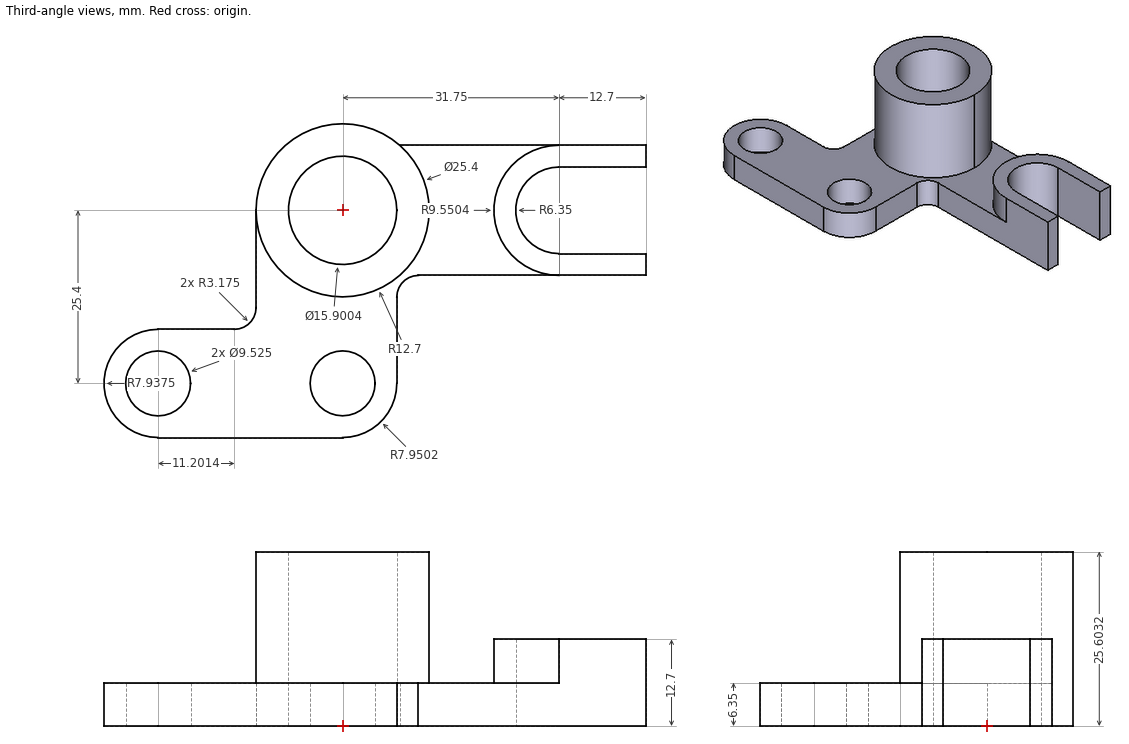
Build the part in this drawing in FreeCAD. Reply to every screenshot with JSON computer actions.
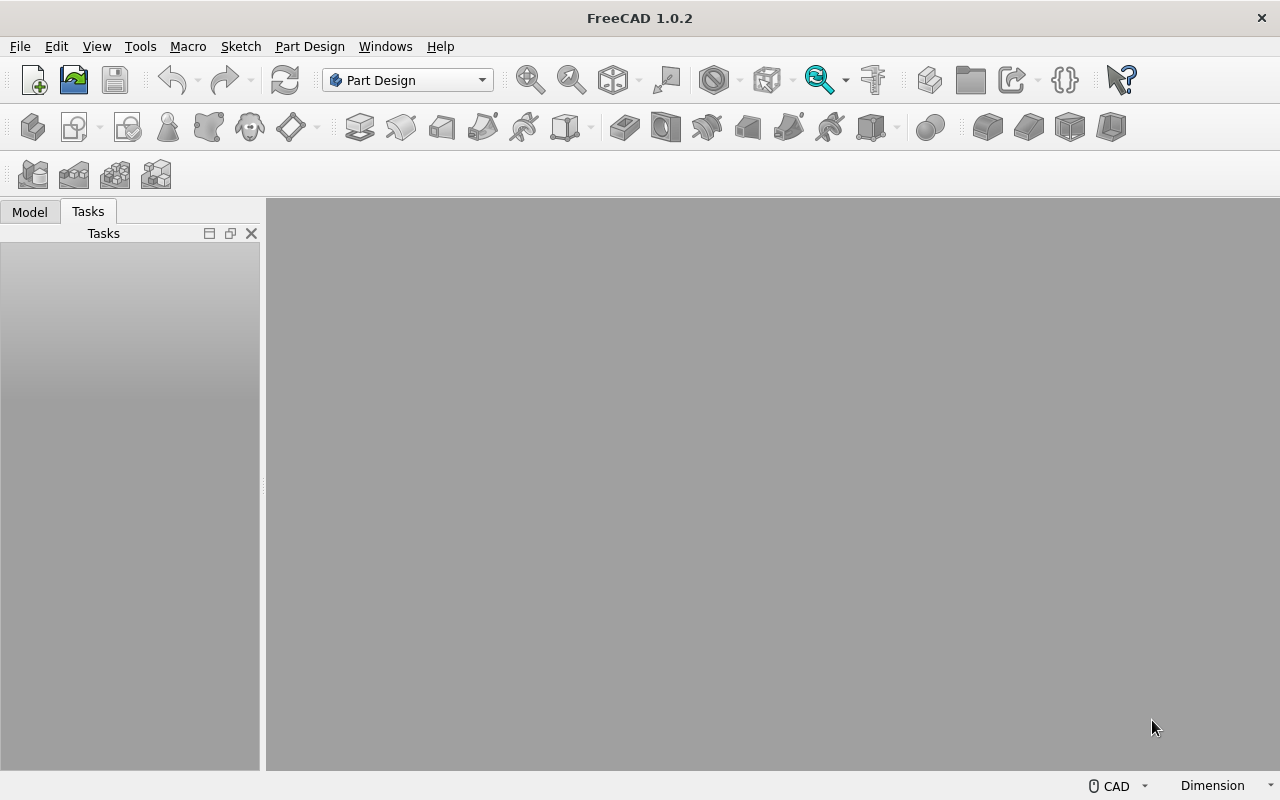
{"action": "left_click", "coordinate": [33, 80]}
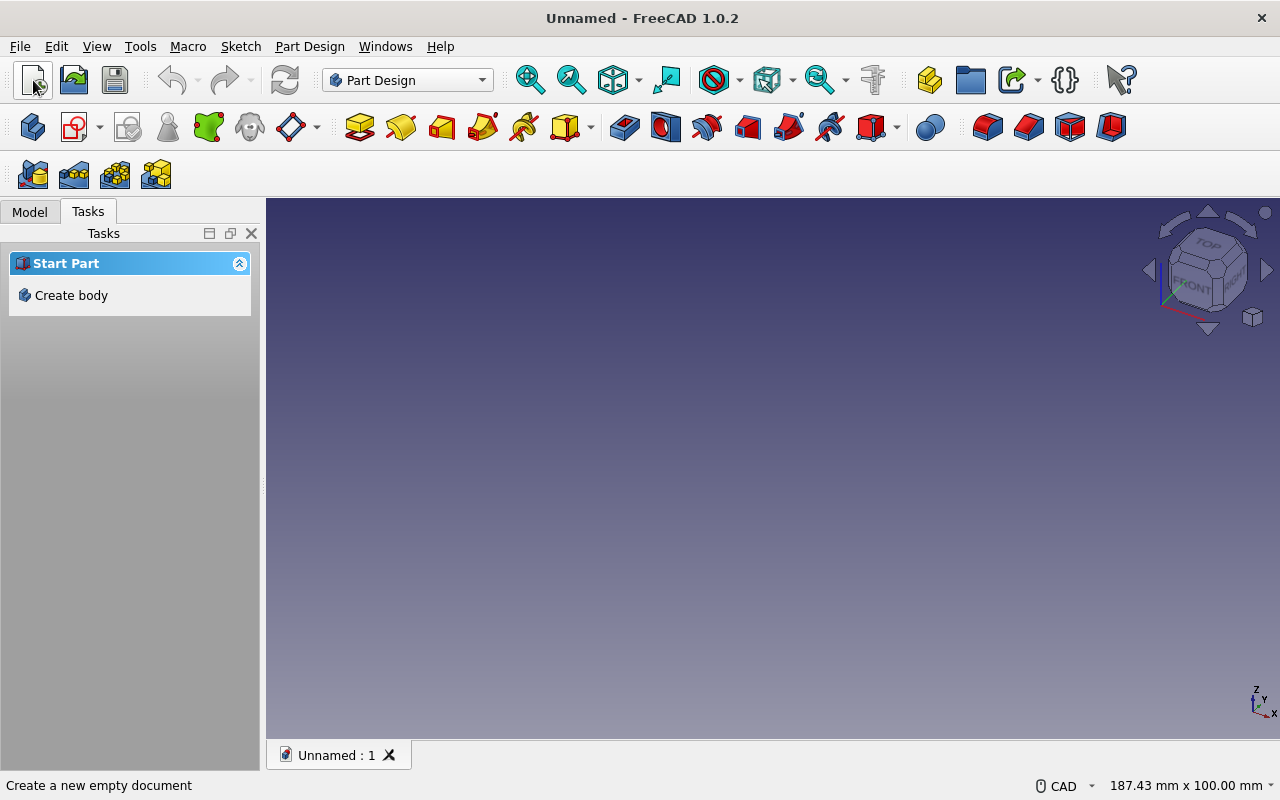
{"action": "left_click", "coordinate": [74, 128]}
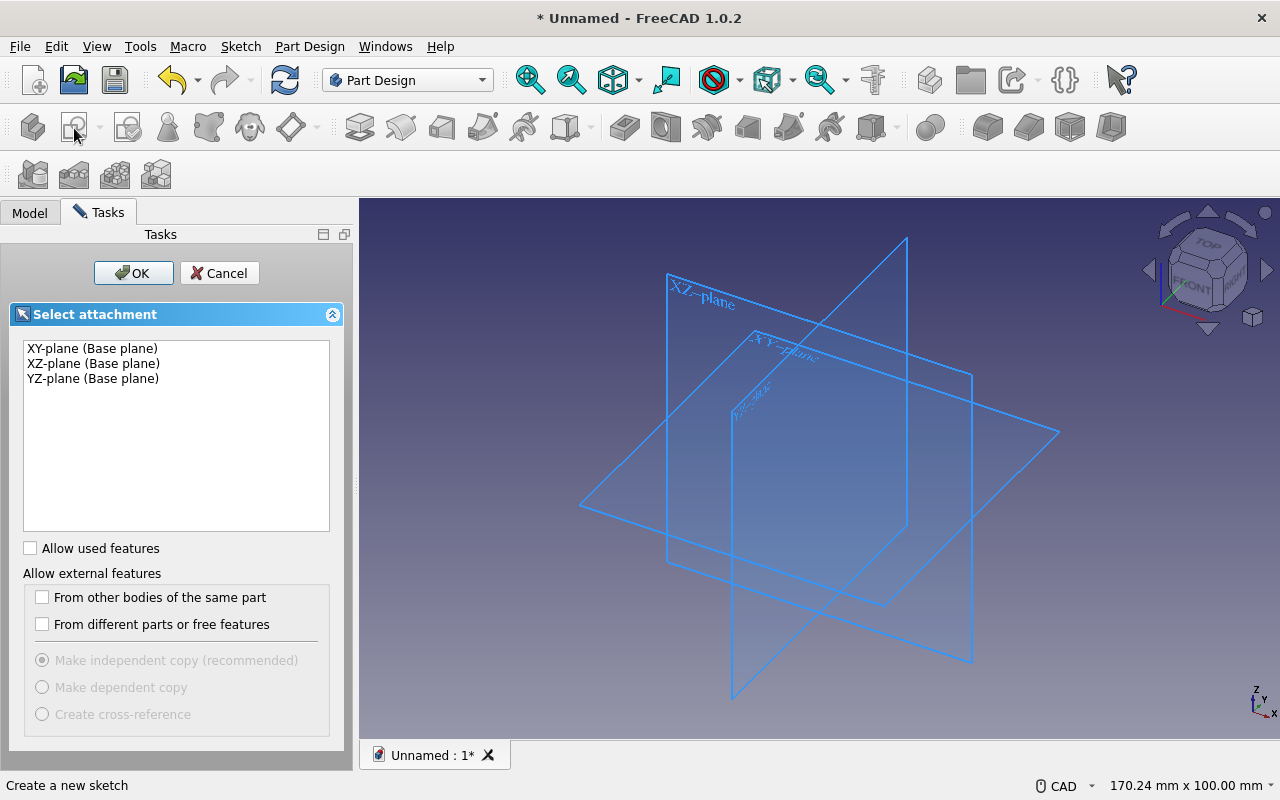
{"action": "left_click", "coordinate": [84, 348]}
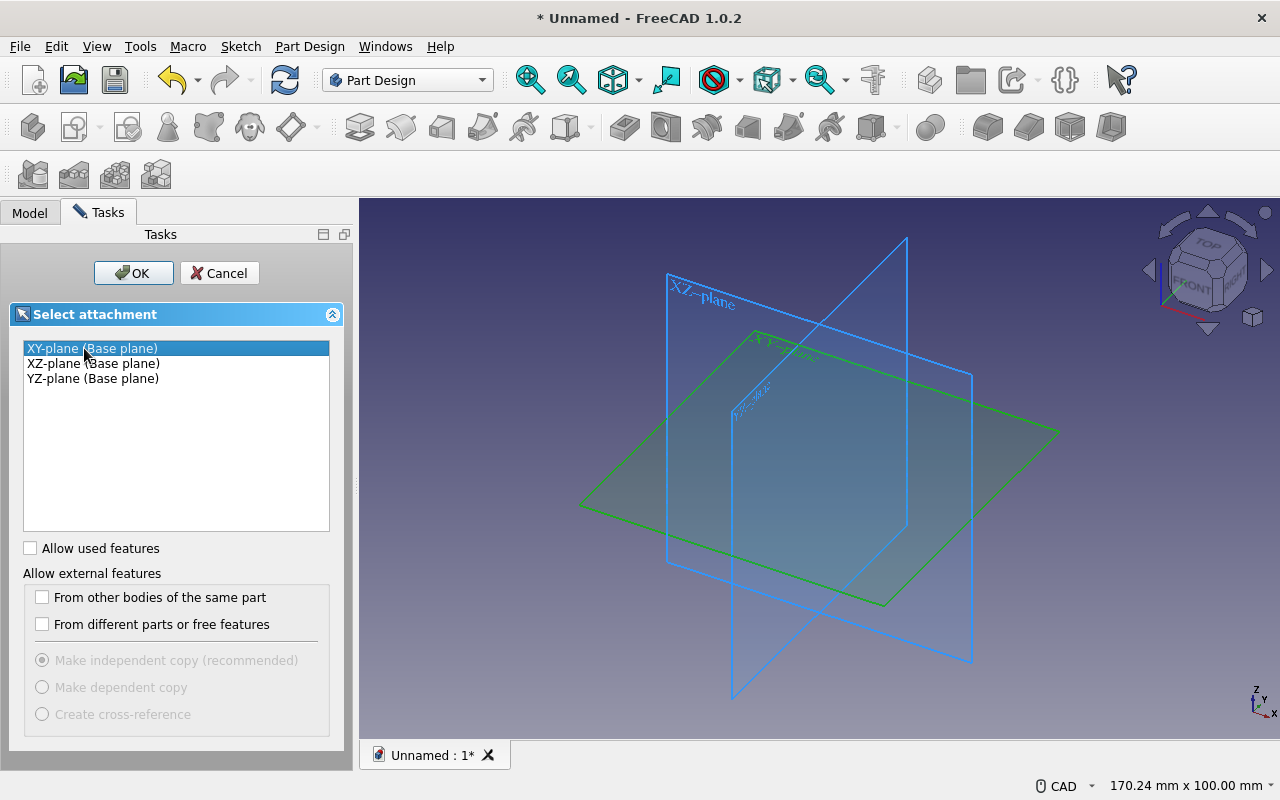
{"action": "left_click", "coordinate": [134, 273]}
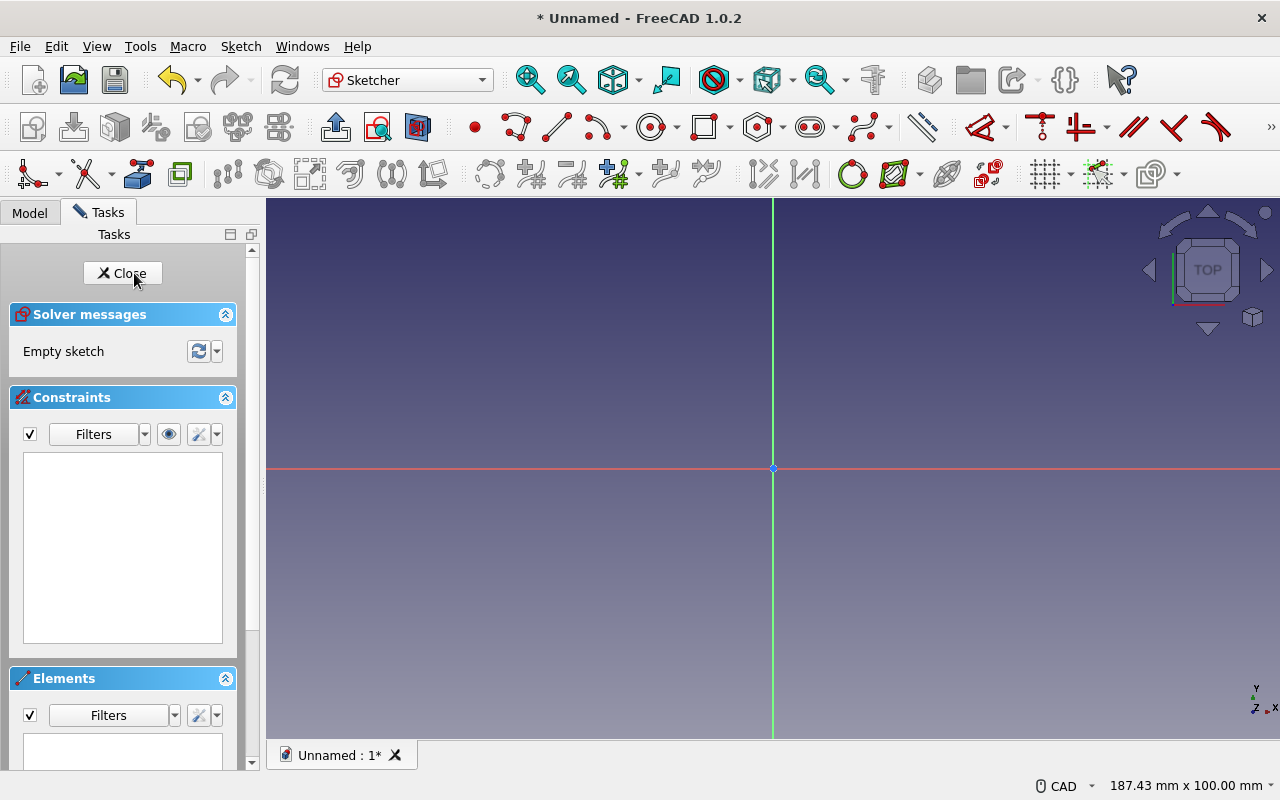
{"action": "scroll", "coordinate": [813, 468], "scroll_direction": "up", "scroll_amount": 5}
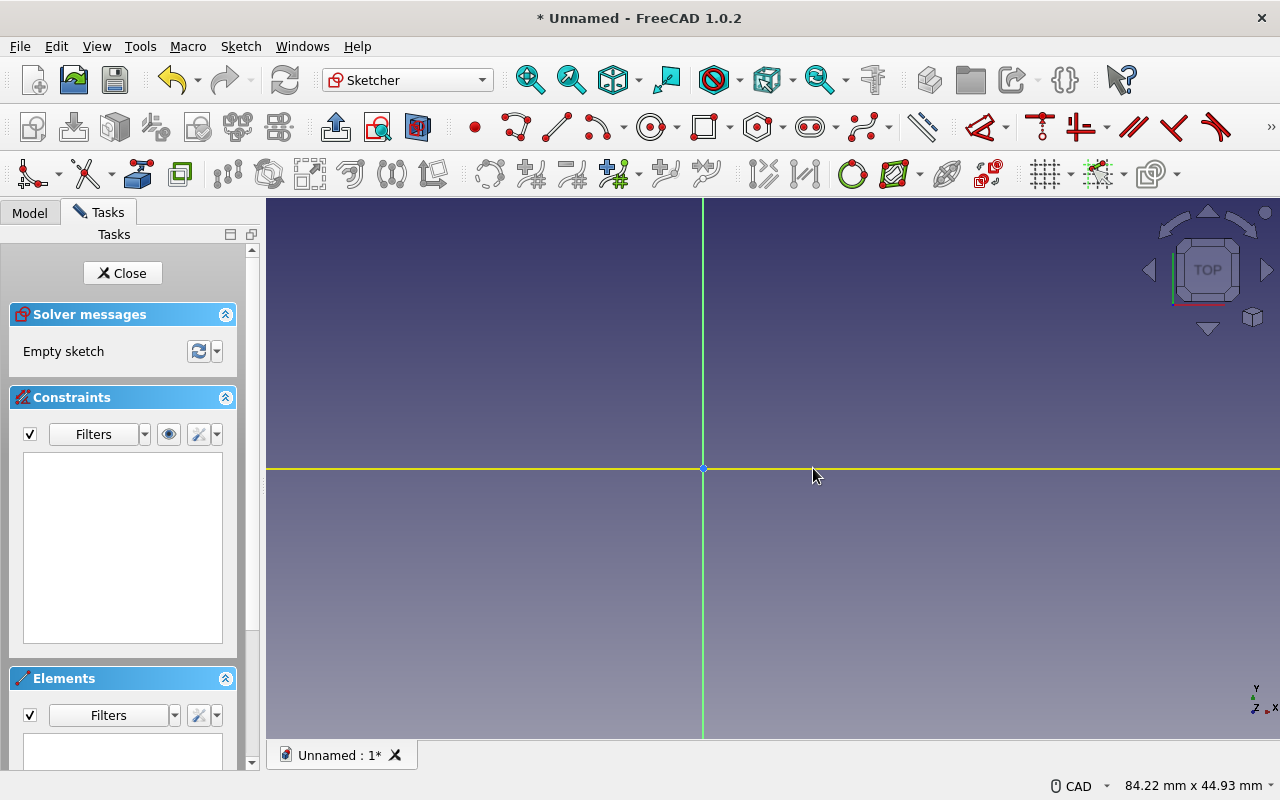
{"action": "left_click", "coordinate": [650, 128]}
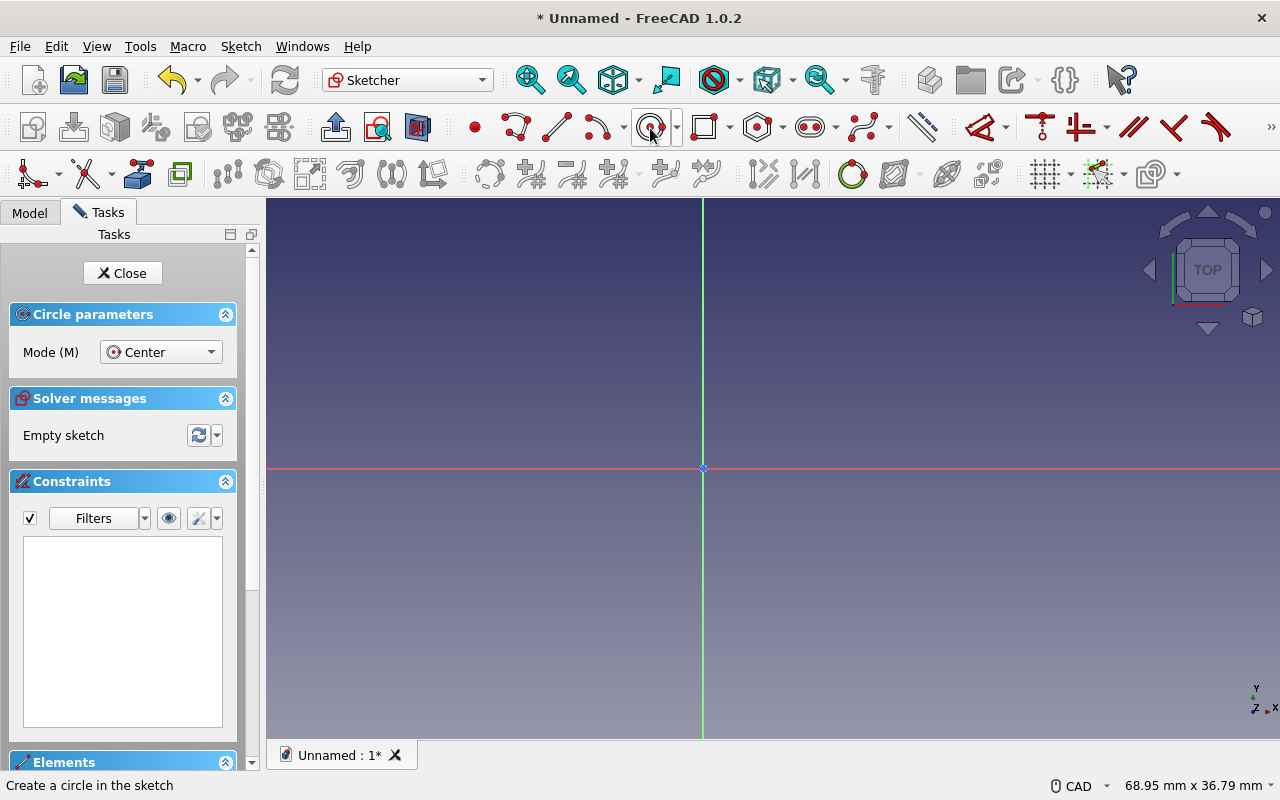
{"action": "left_click", "coordinate": [703, 468]}
{"action": "left_click", "coordinate": [835, 336]}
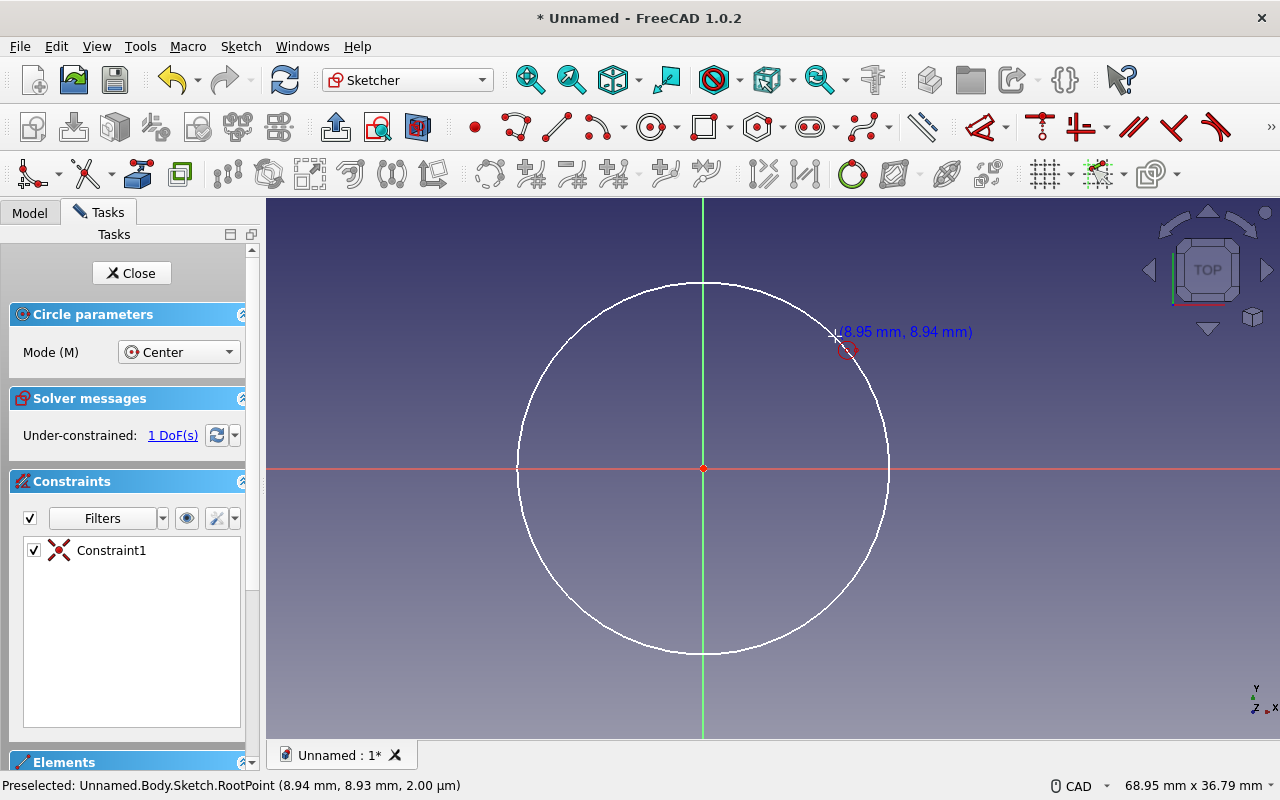
{"action": "left_click", "coordinate": [703, 468]}
{"action": "left_click", "coordinate": [786, 386]}
{"action": "key", "text": "Escape"}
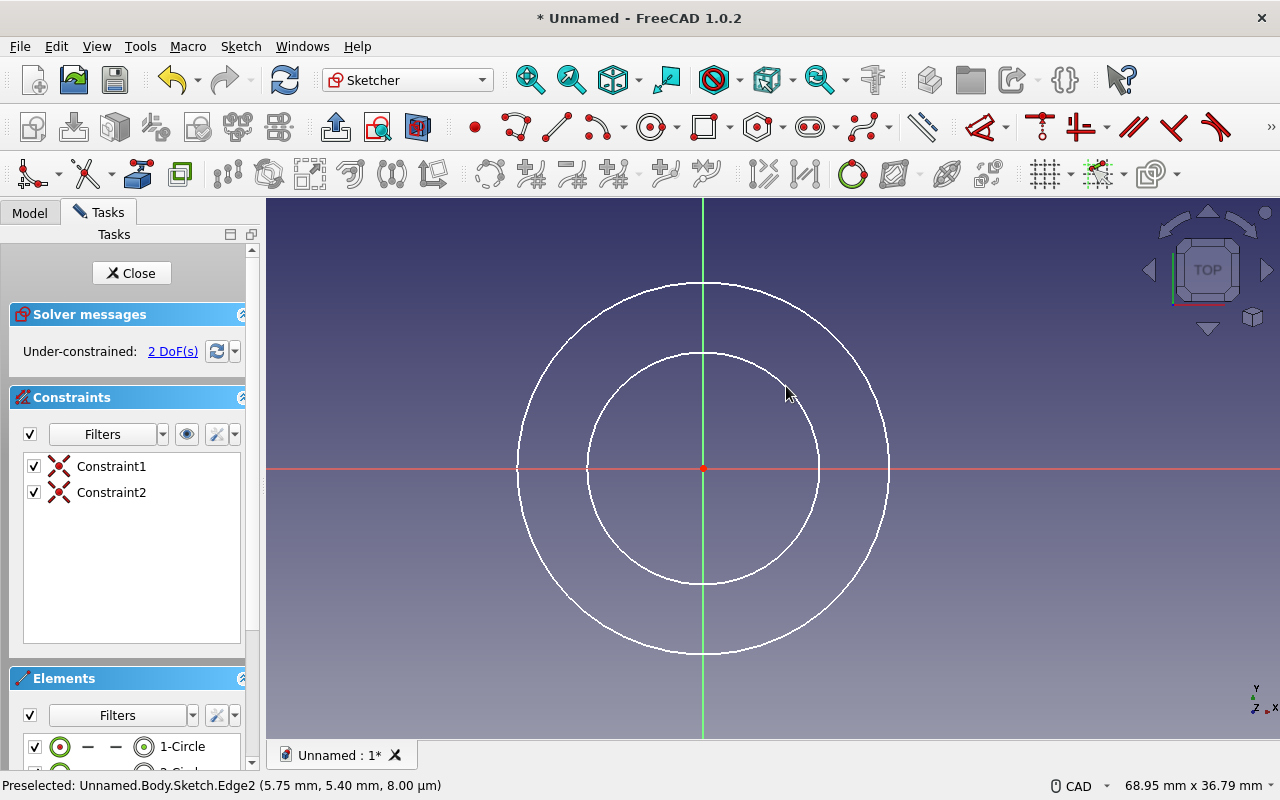
{"action": "left_click", "coordinate": [980, 128]}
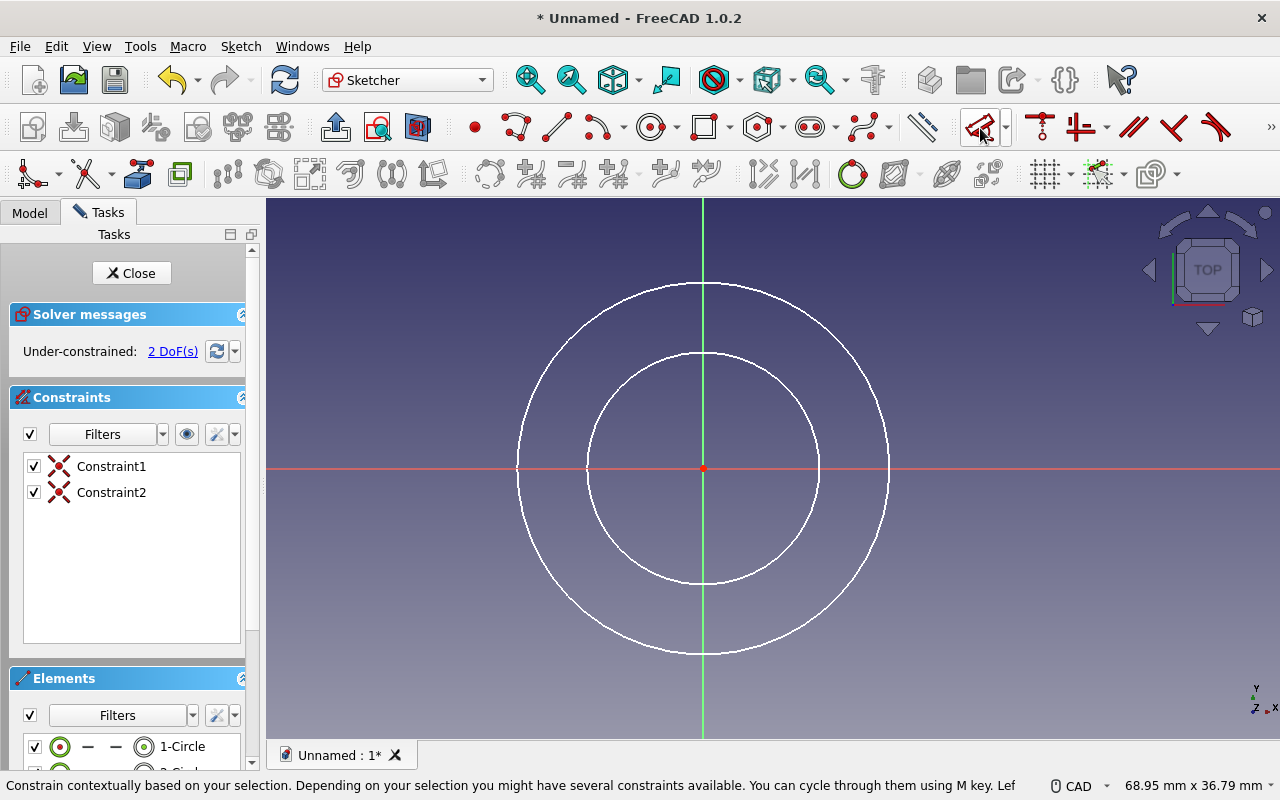
{"action": "left_click", "coordinate": [835, 337]}
{"action": "left_click", "coordinate": [858, 314]}